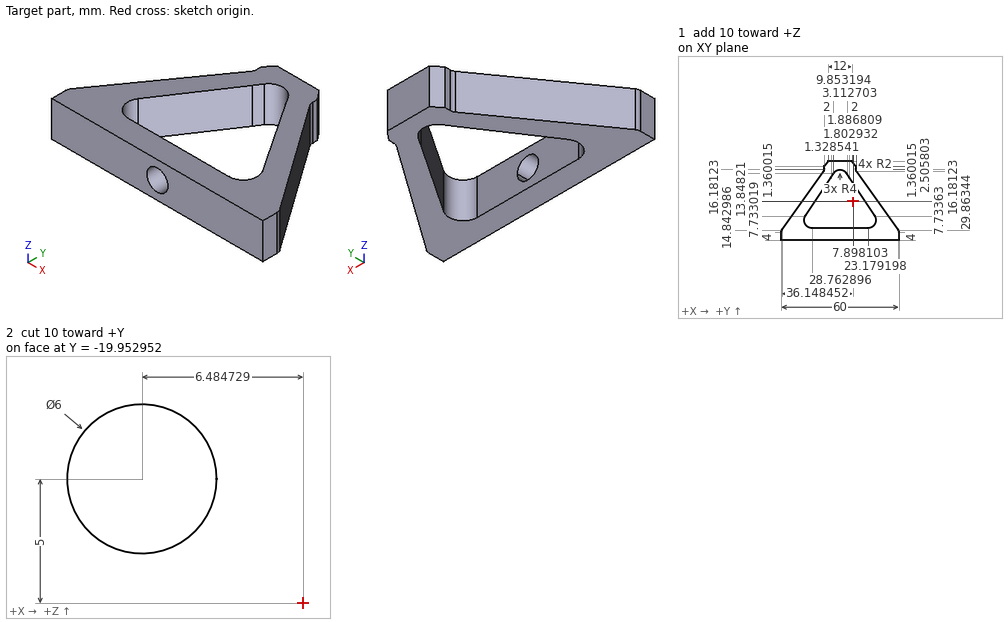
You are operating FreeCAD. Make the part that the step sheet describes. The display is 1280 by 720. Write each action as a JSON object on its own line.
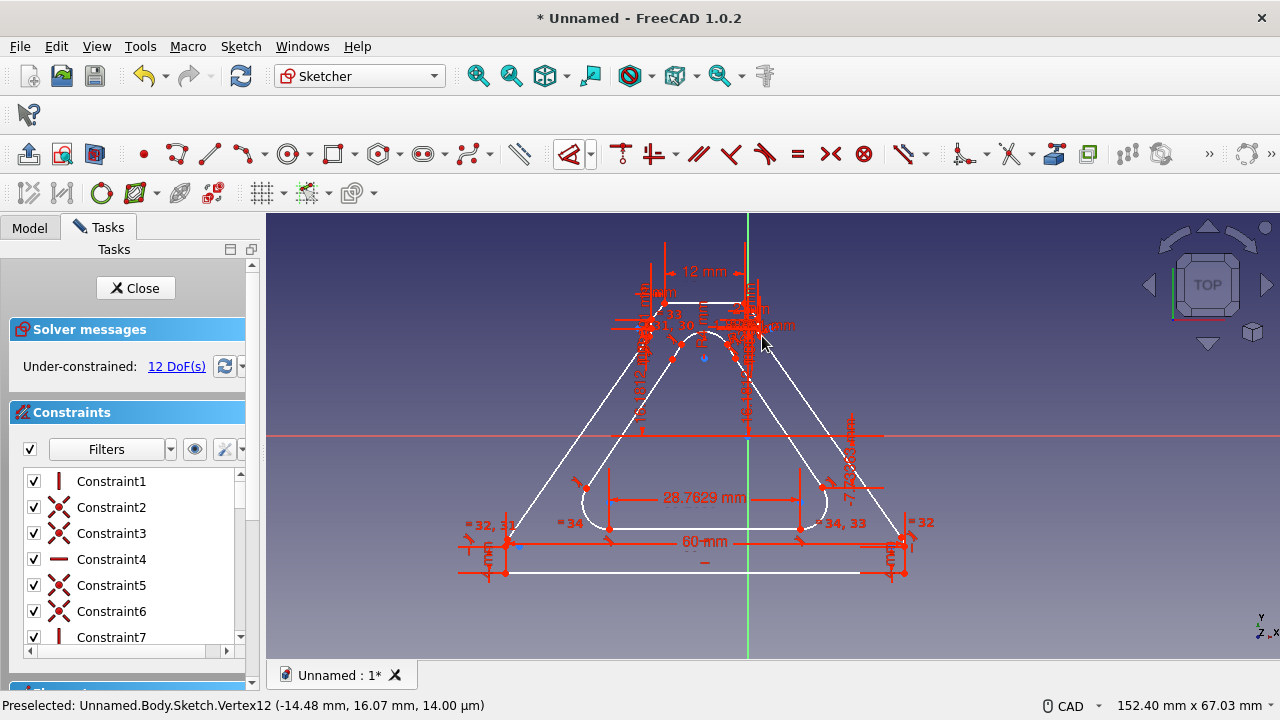
{"action": "left_click", "coordinate": [587, 488]}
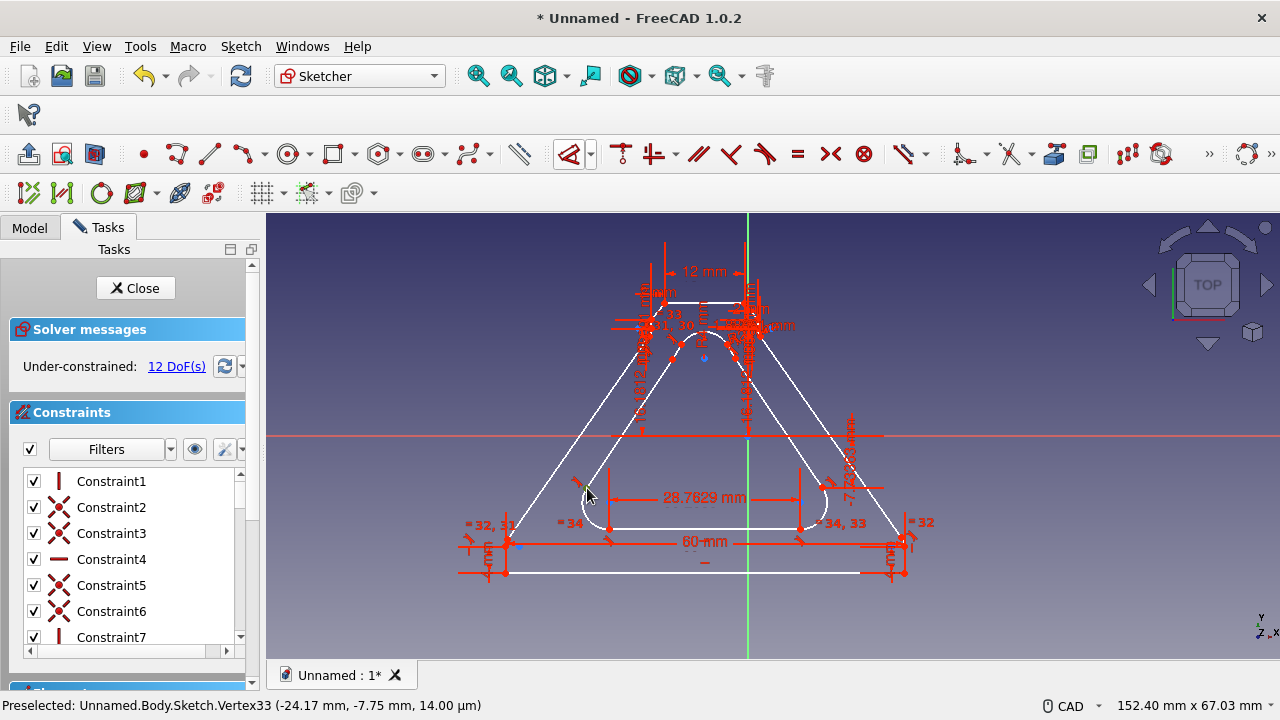
{"action": "left_click", "coordinate": [590, 154]}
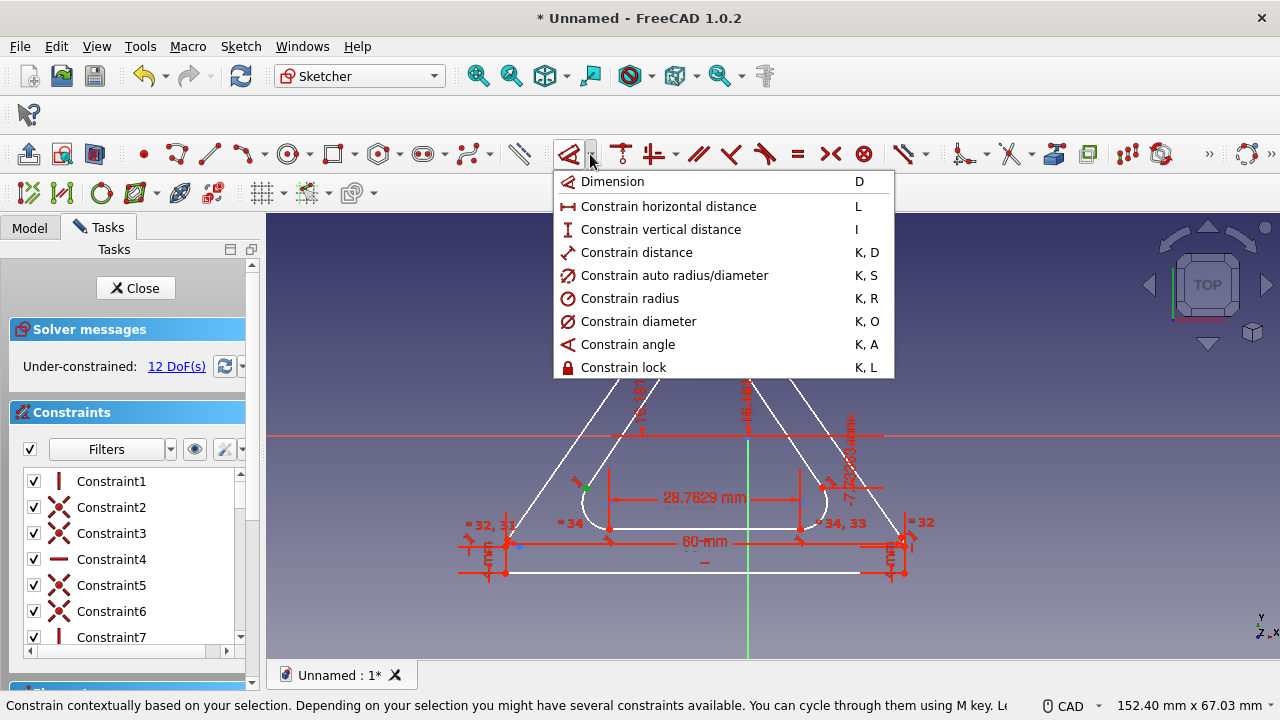
{"action": "left_click", "coordinate": [724, 230]}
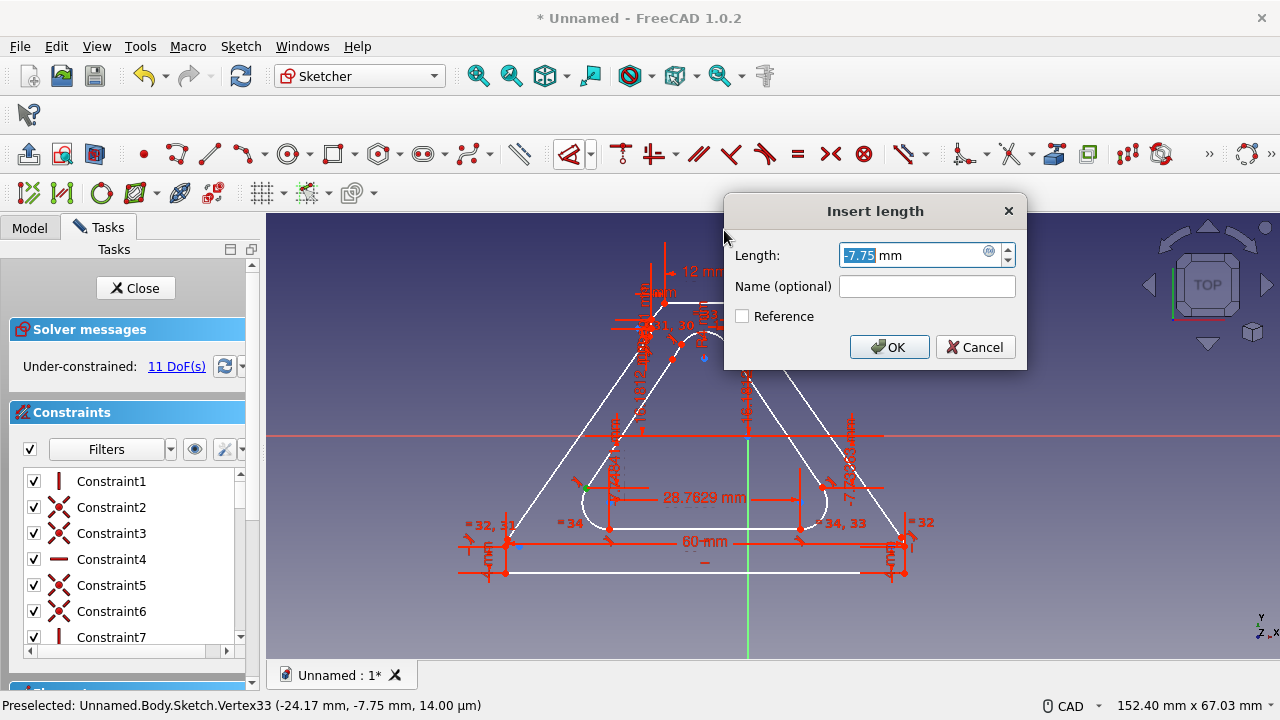
{"action": "type", "text": "-7.733019"}
{"action": "key", "text": "Return"}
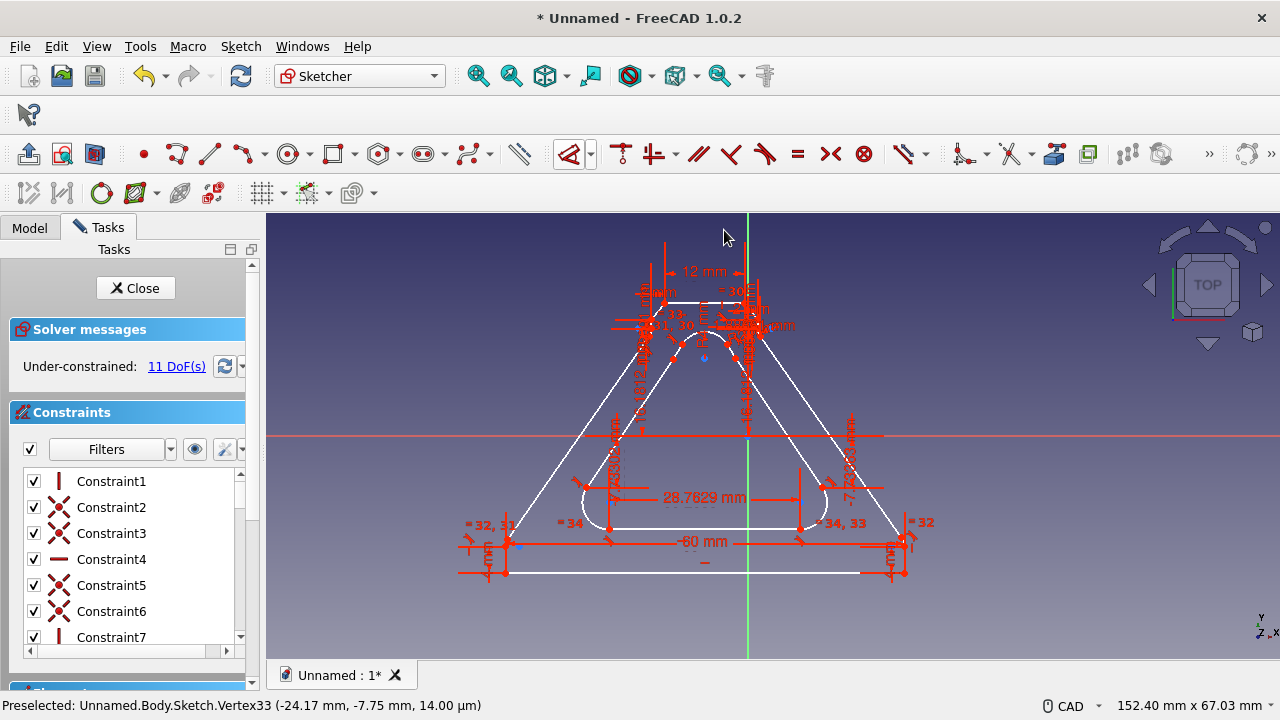
{"action": "left_click", "coordinate": [682, 345]}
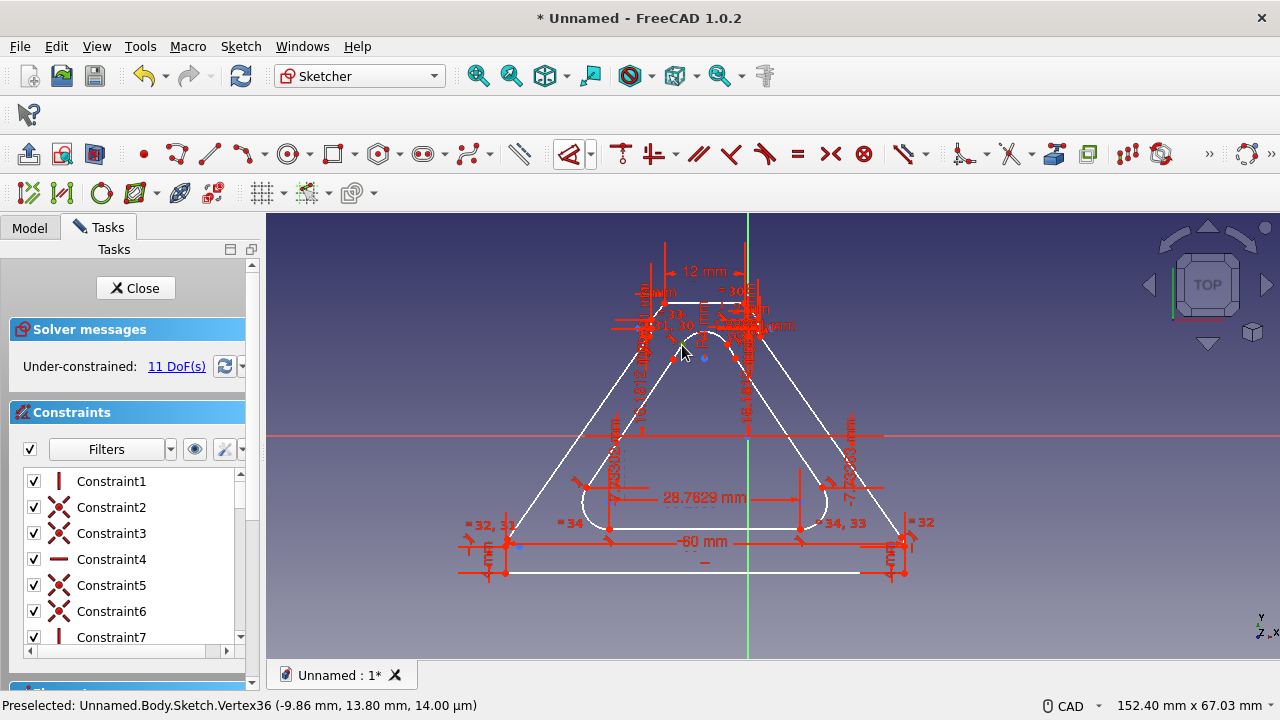
{"action": "left_click", "coordinate": [590, 154]}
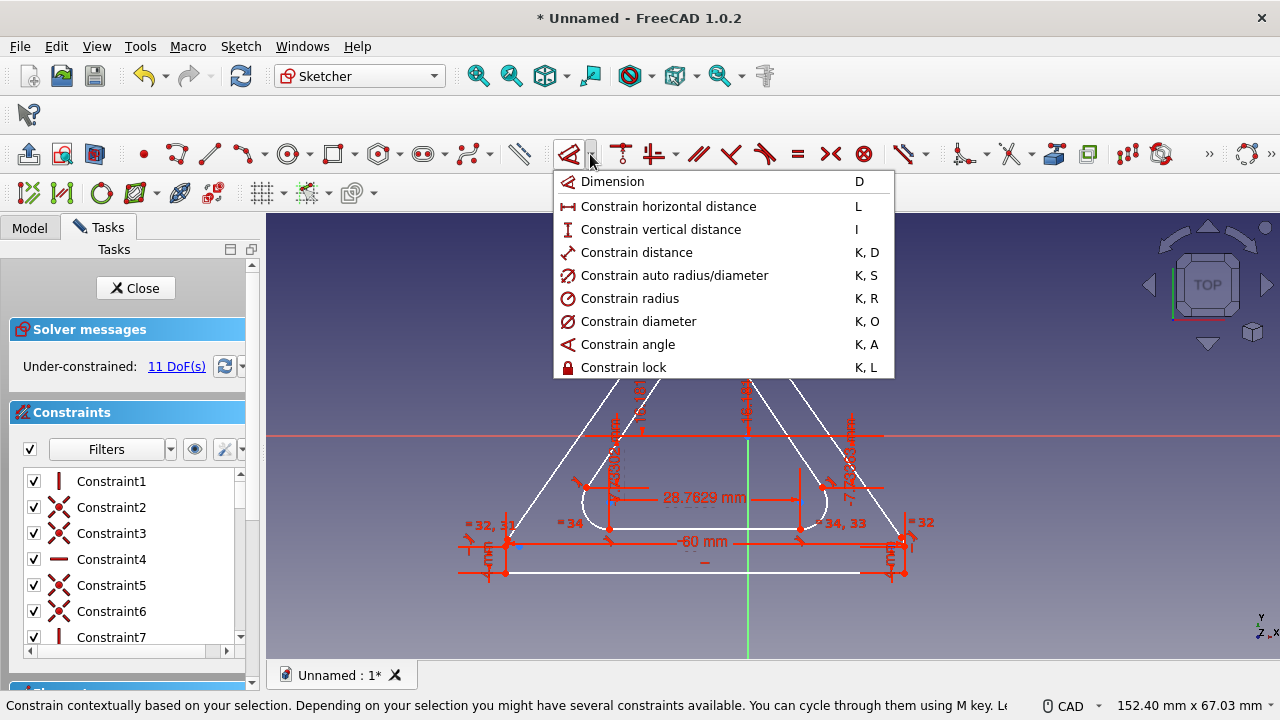
{"action": "left_click", "coordinate": [724, 206]}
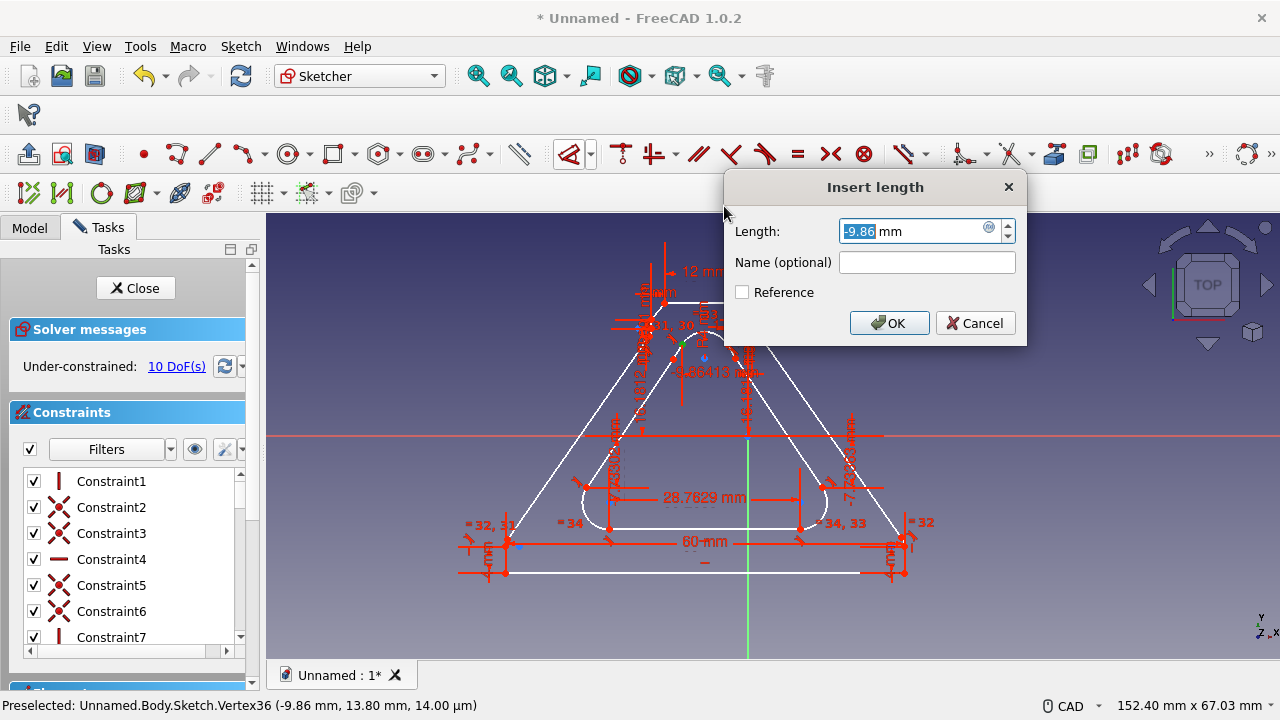
{"action": "type", "text": "-9.853194"}
{"action": "key", "text": "Return"}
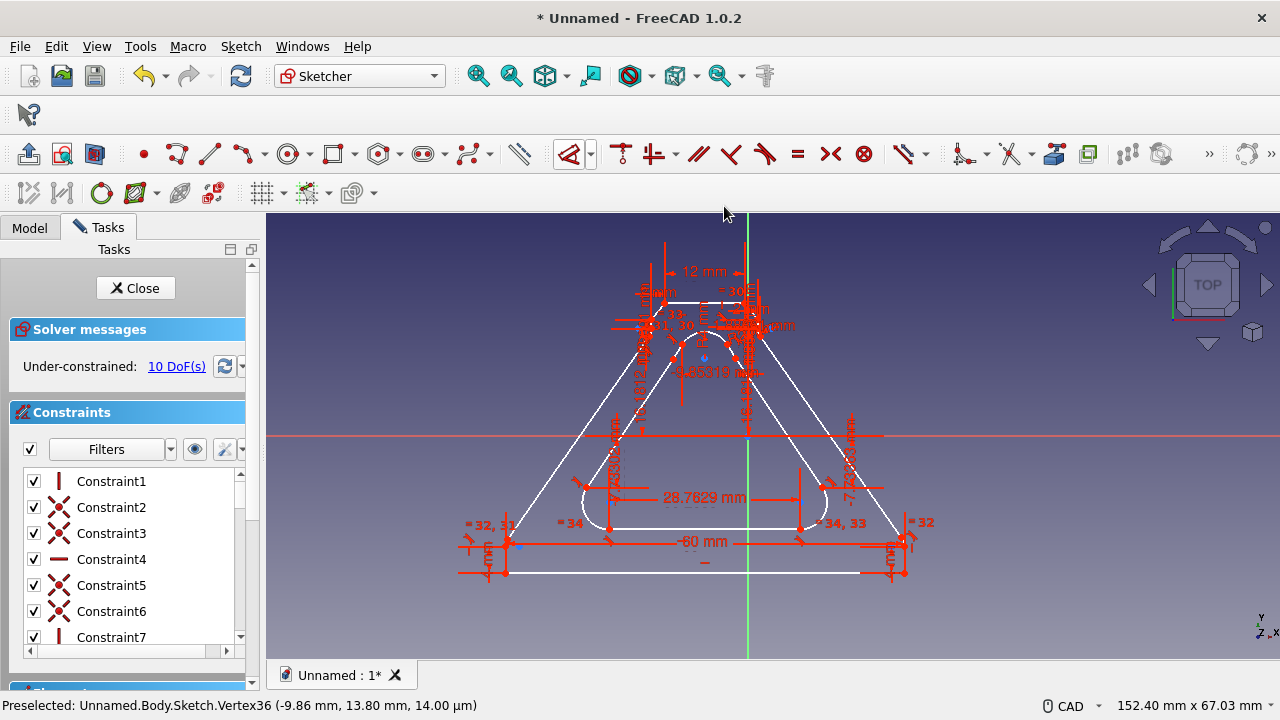
{"action": "left_click", "coordinate": [682, 345]}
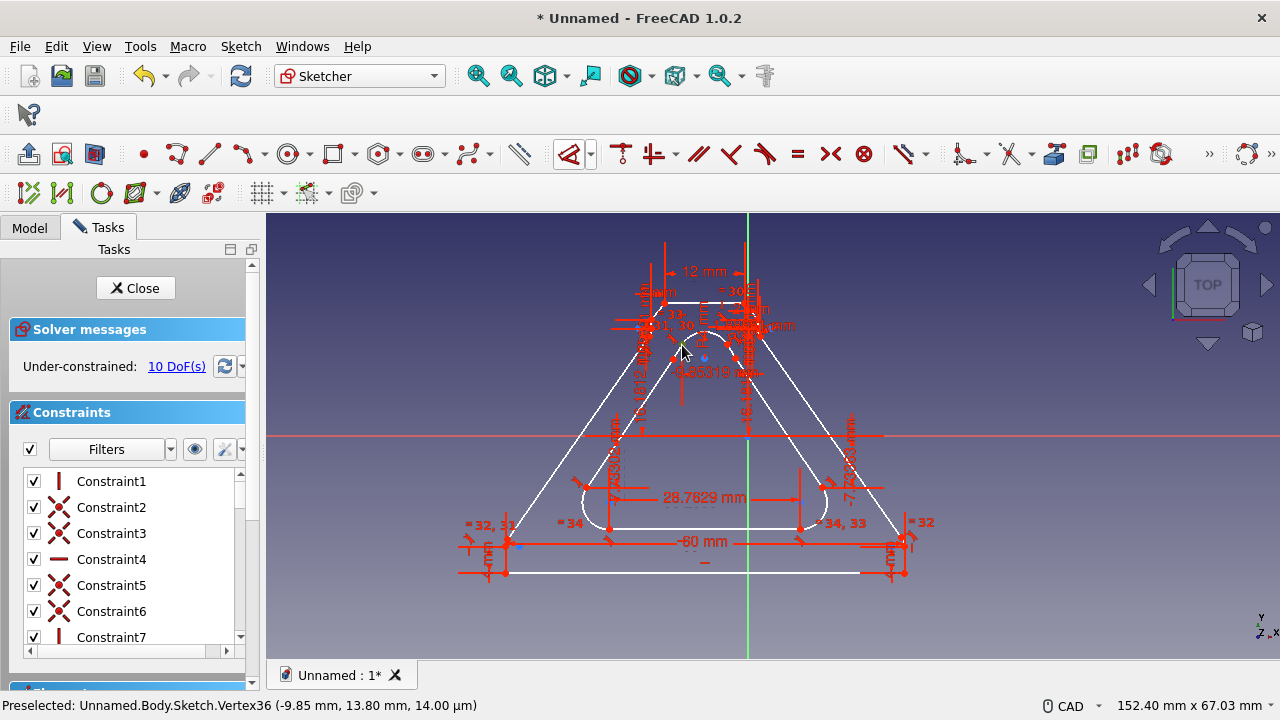
{"action": "left_click", "coordinate": [590, 154]}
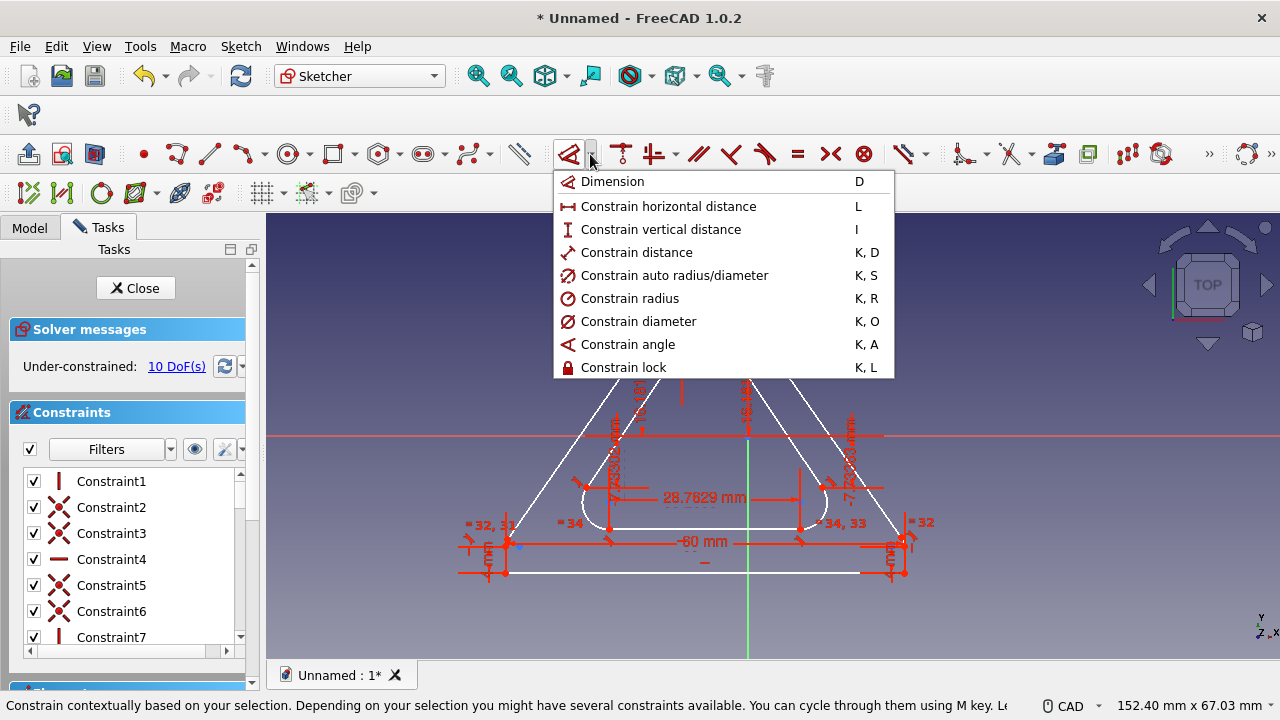
{"action": "left_click", "coordinate": [724, 230]}